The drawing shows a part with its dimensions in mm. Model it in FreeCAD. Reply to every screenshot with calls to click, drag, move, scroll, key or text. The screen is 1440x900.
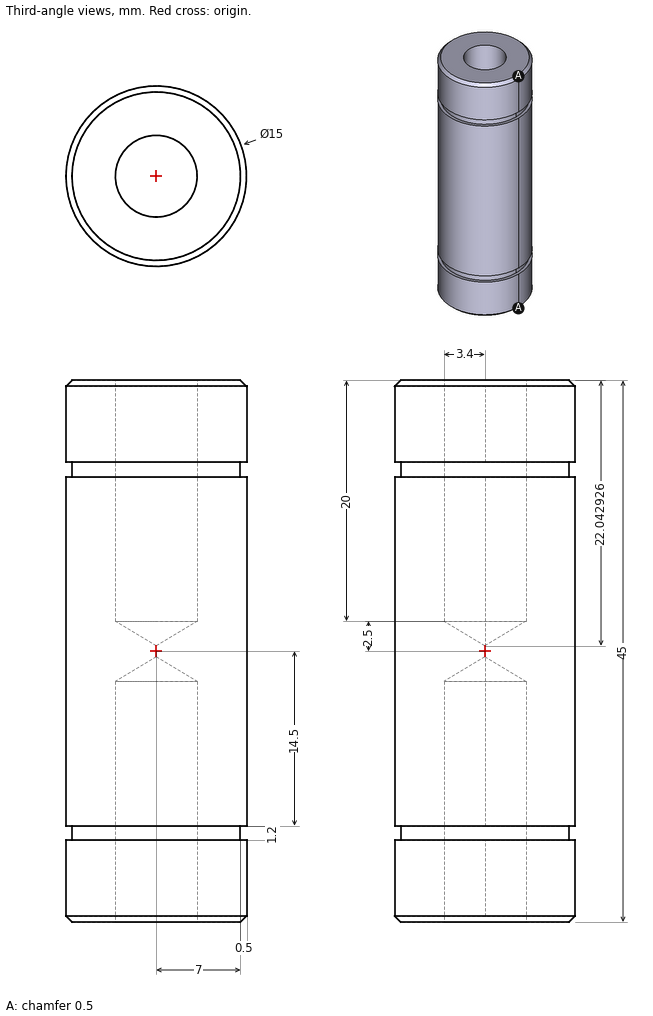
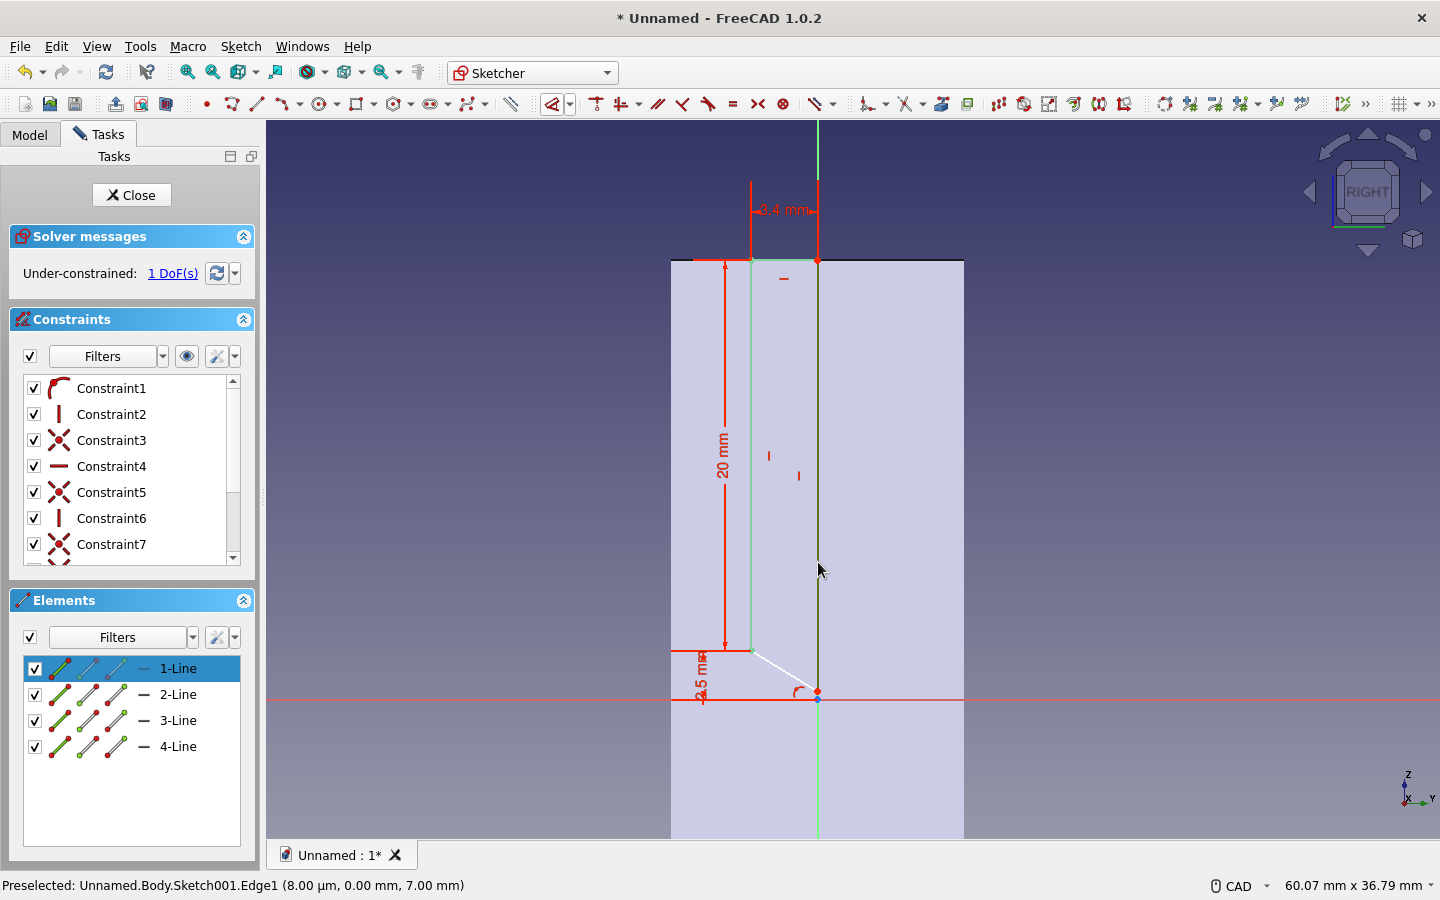
click(570, 104)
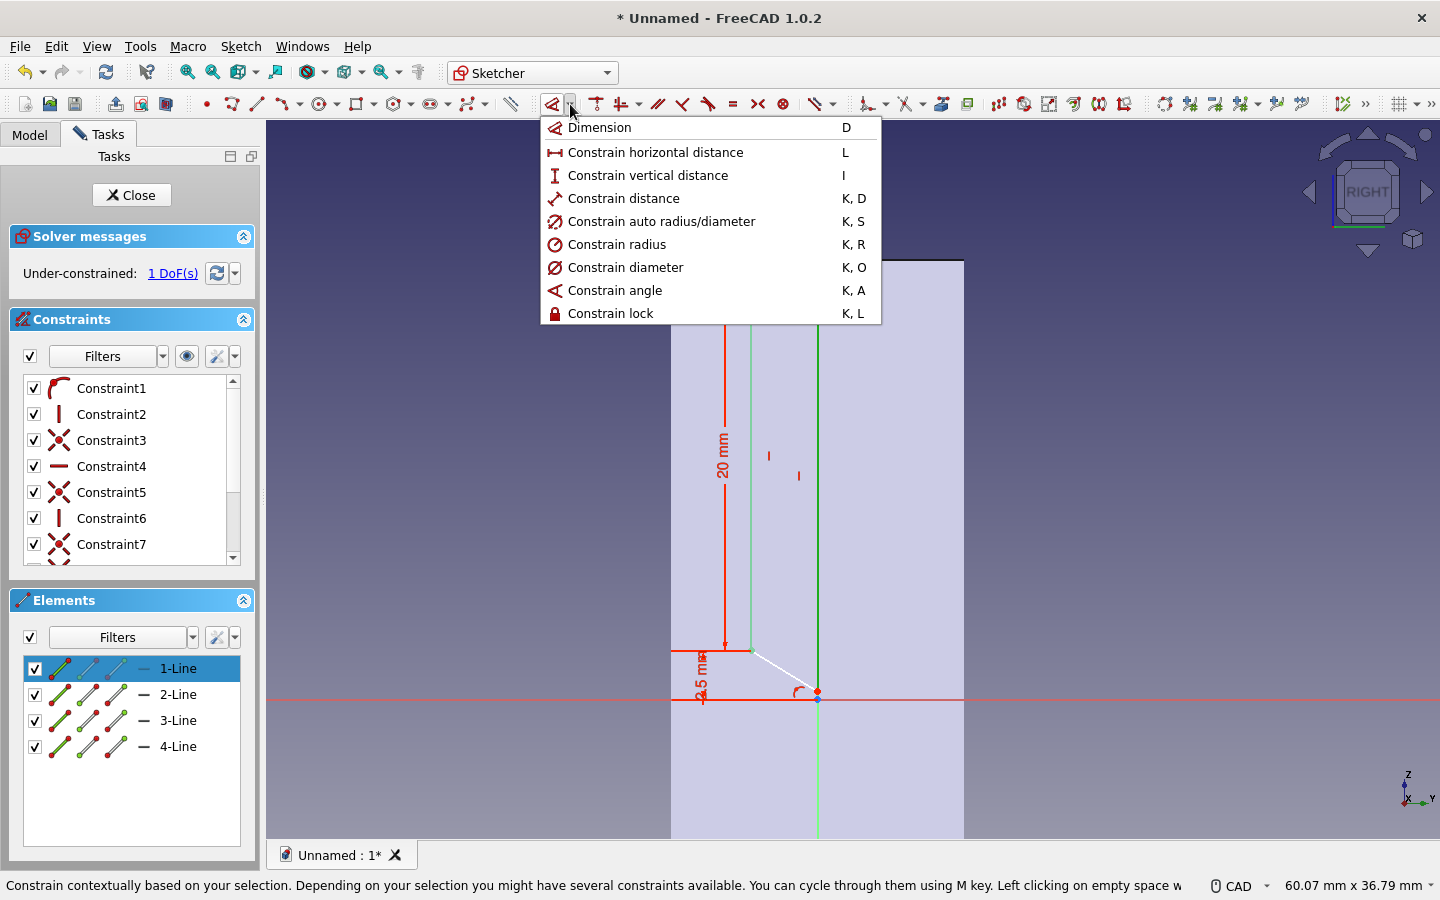
click(711, 176)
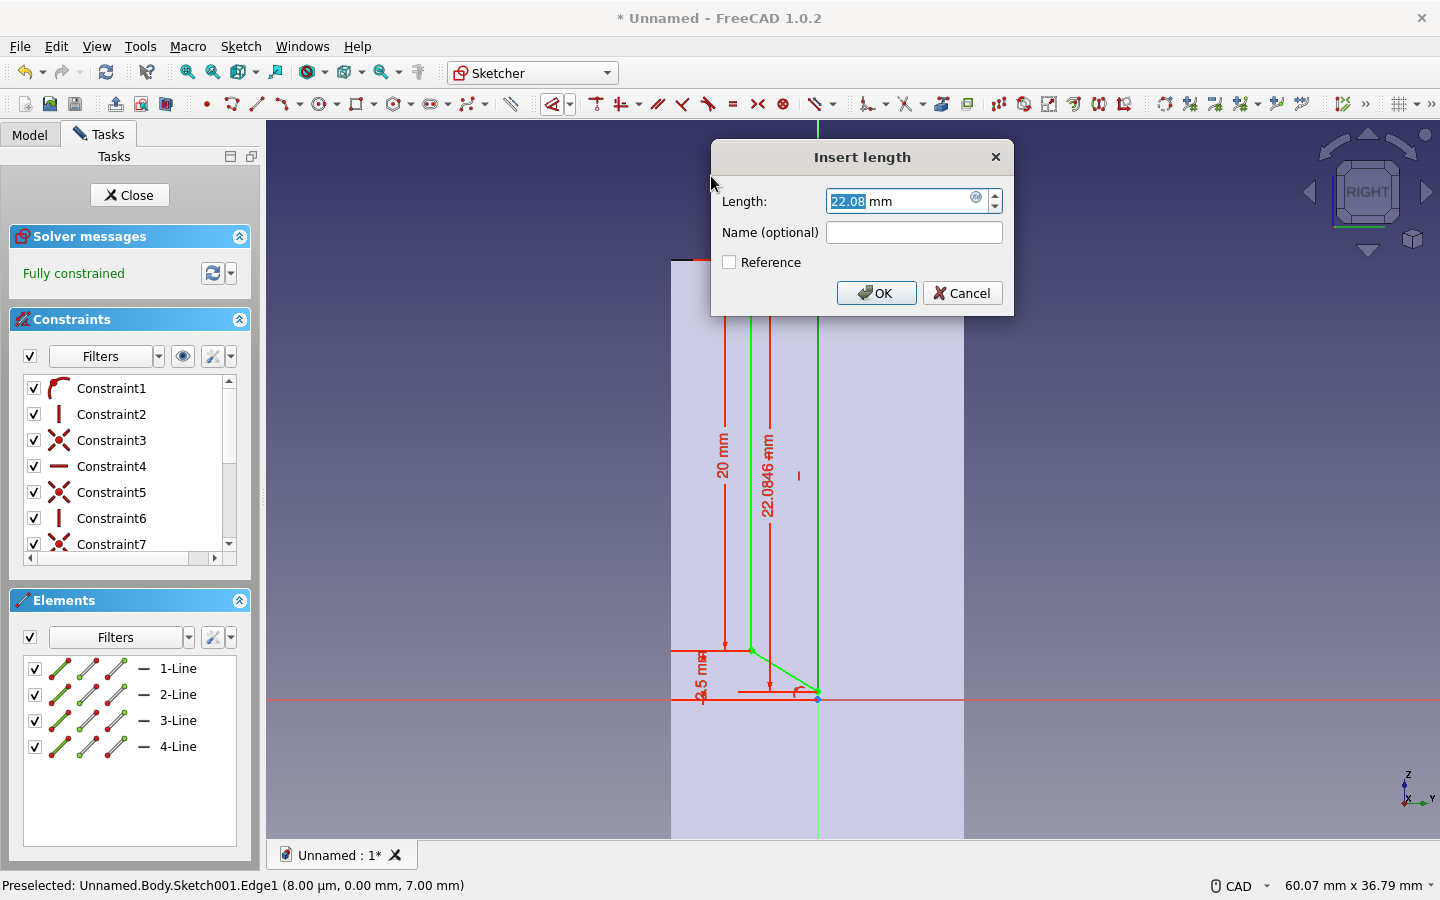
text(22.042926)
key(Return)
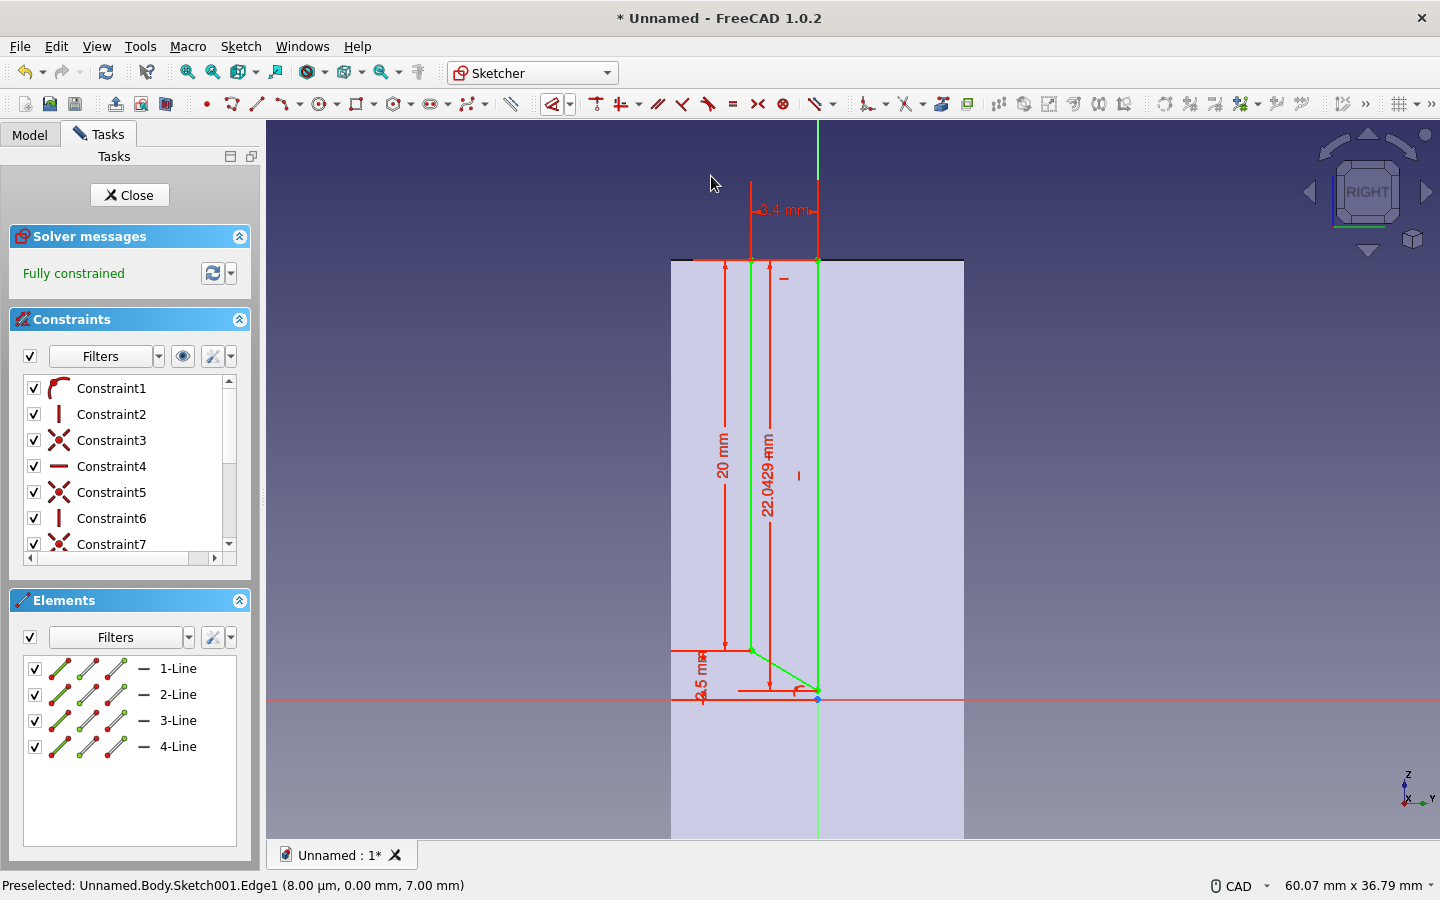
click(130, 195)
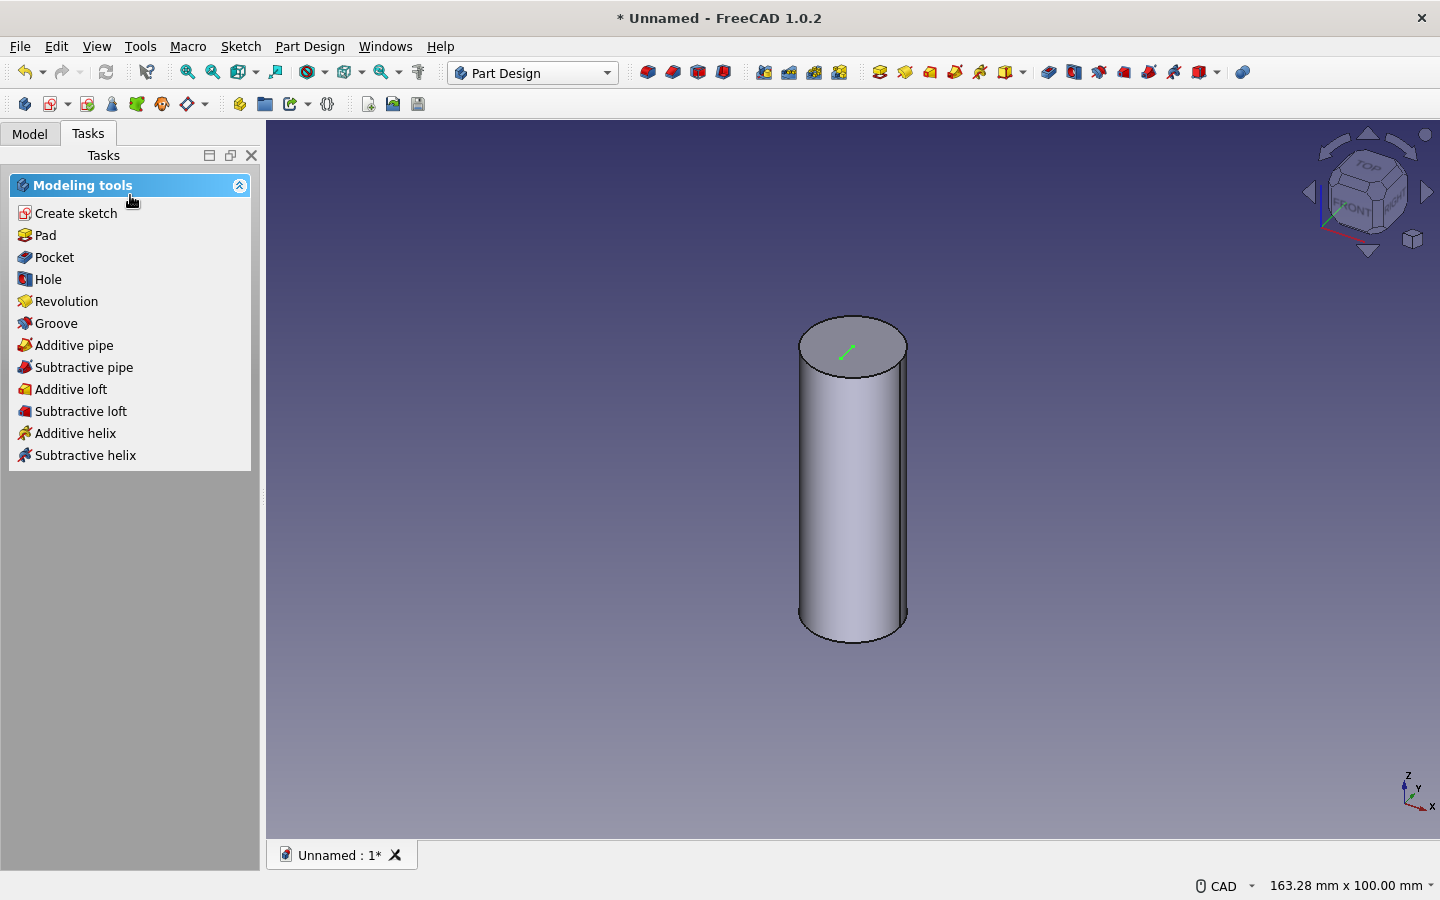
click(1099, 72)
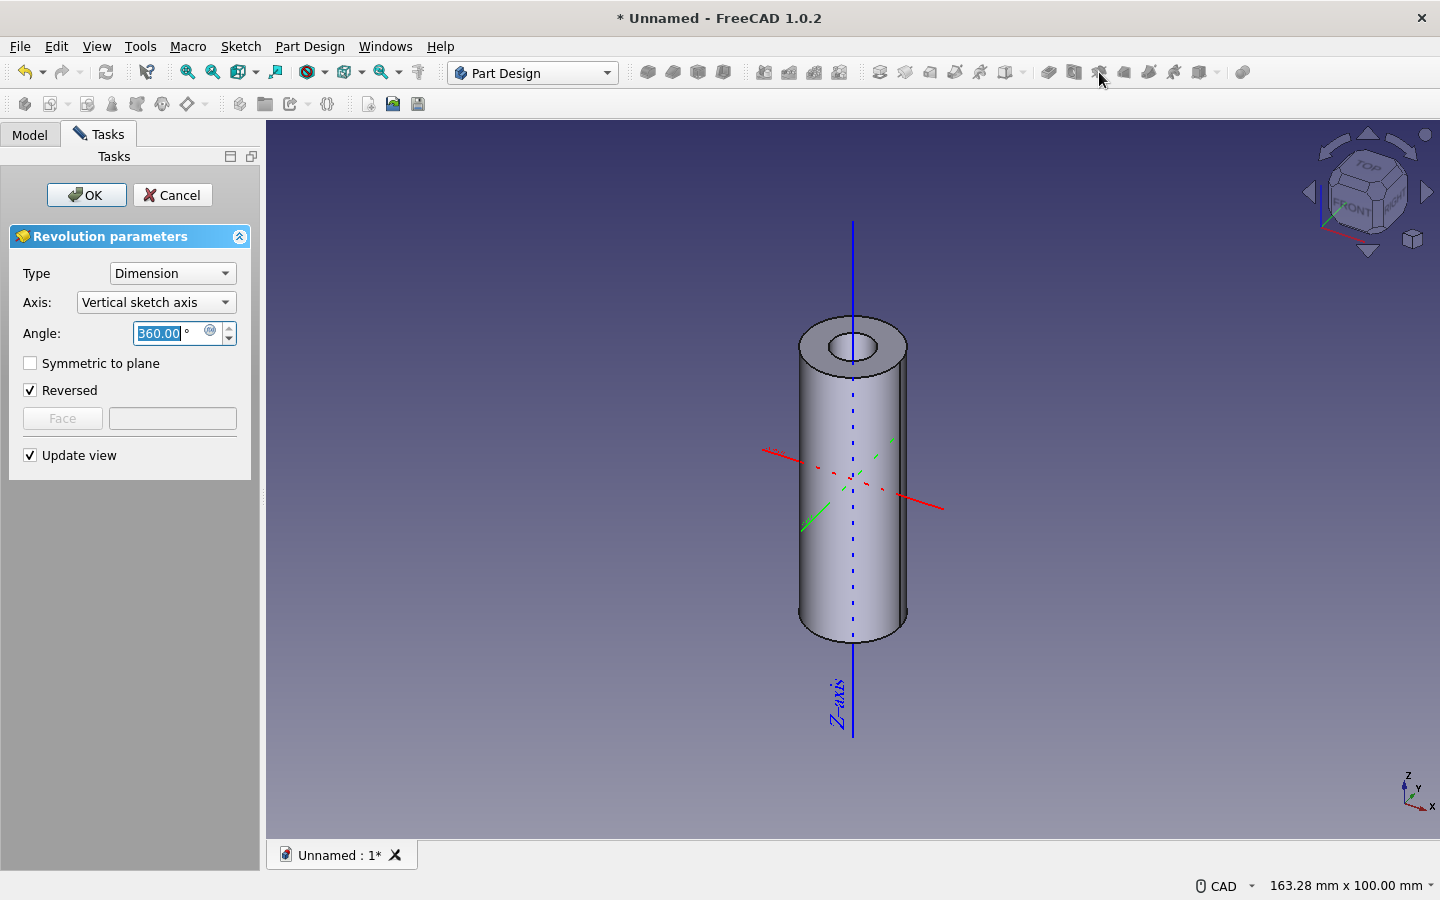
click(87, 195)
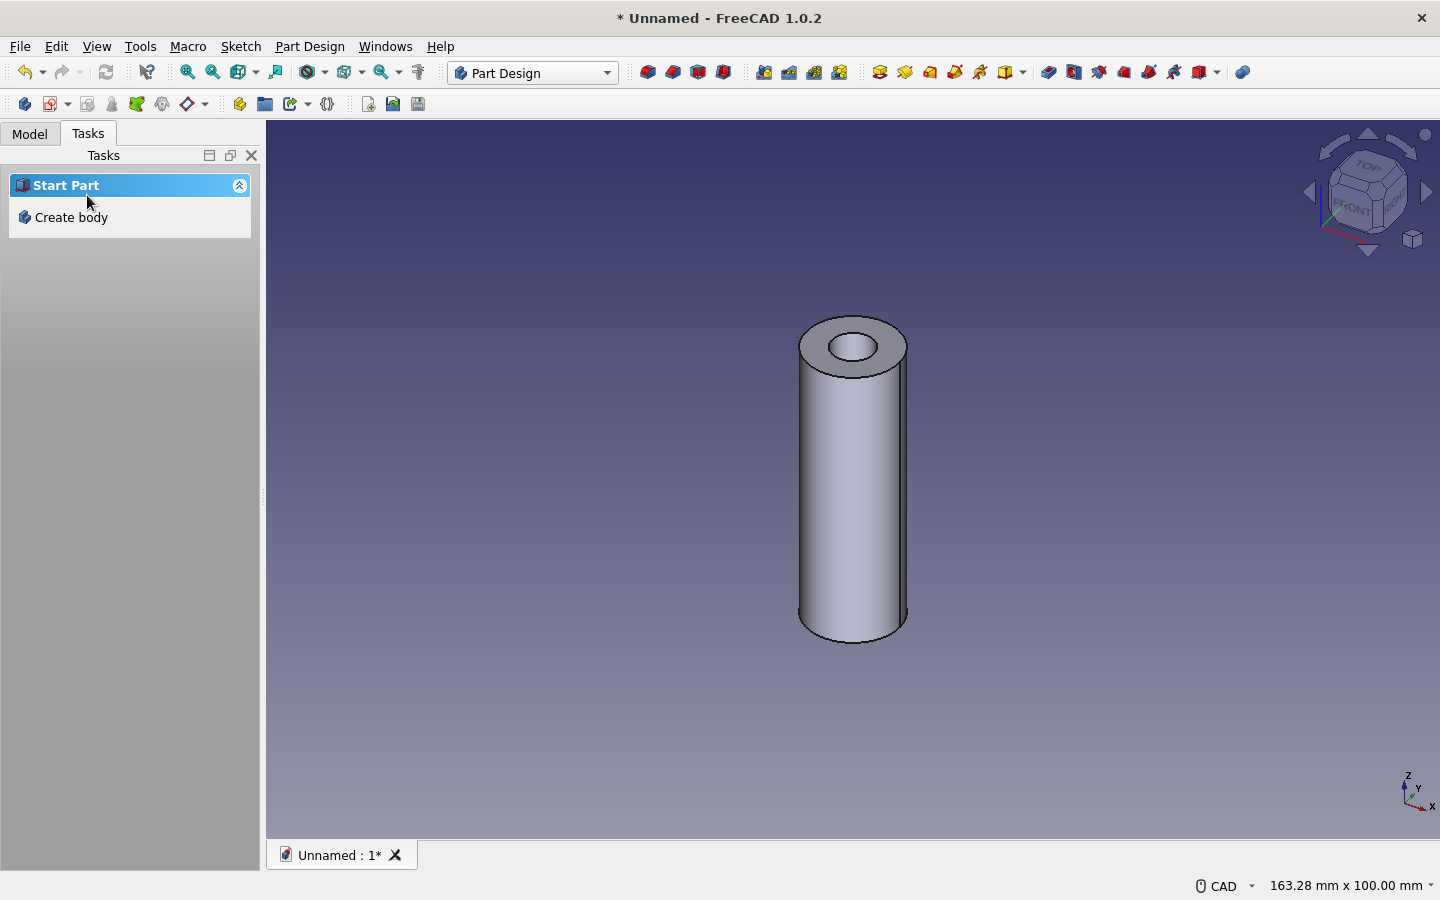
click(869, 641)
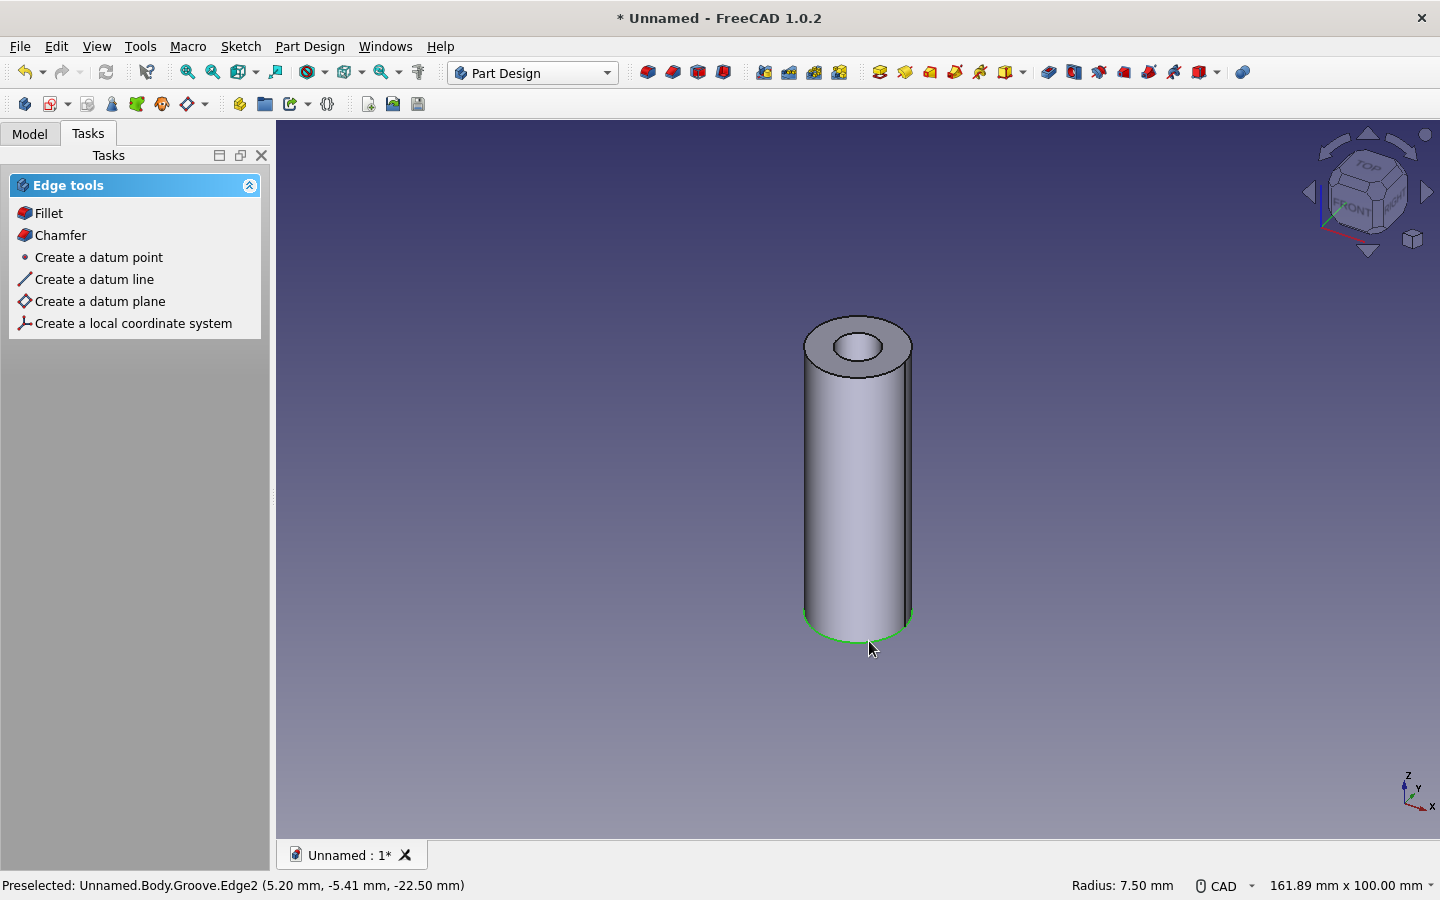
click(811, 331, ctrl)